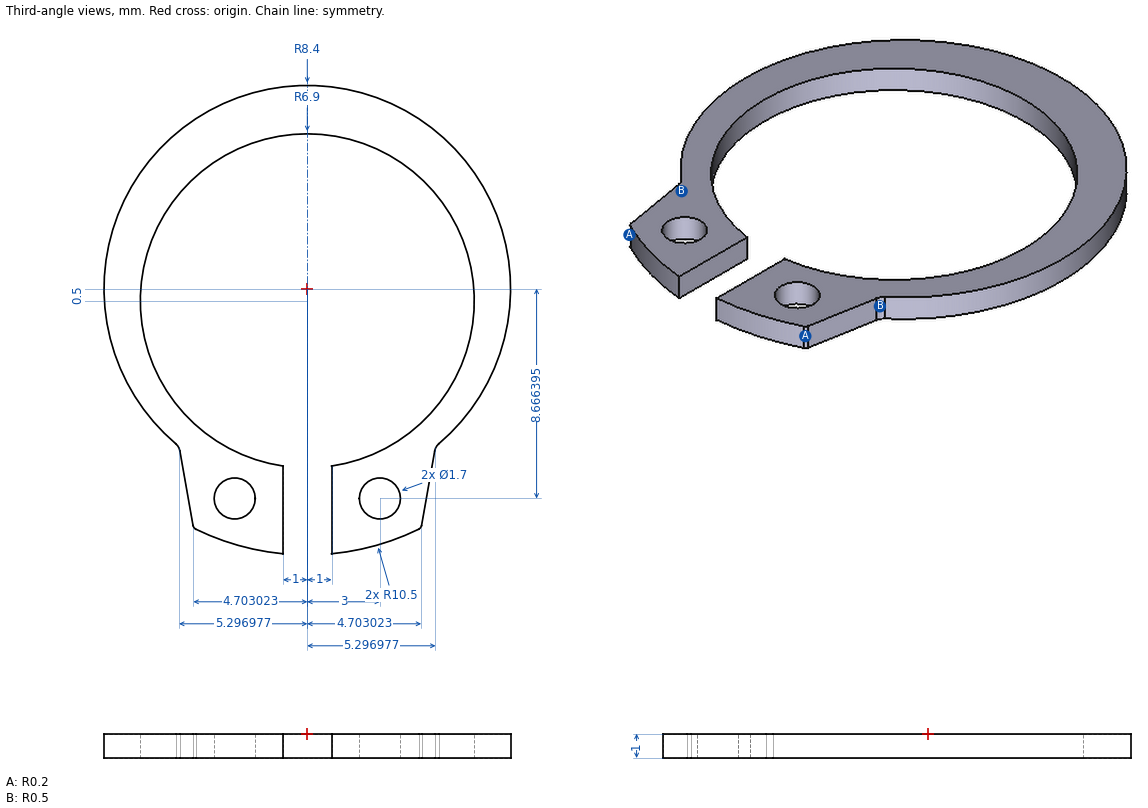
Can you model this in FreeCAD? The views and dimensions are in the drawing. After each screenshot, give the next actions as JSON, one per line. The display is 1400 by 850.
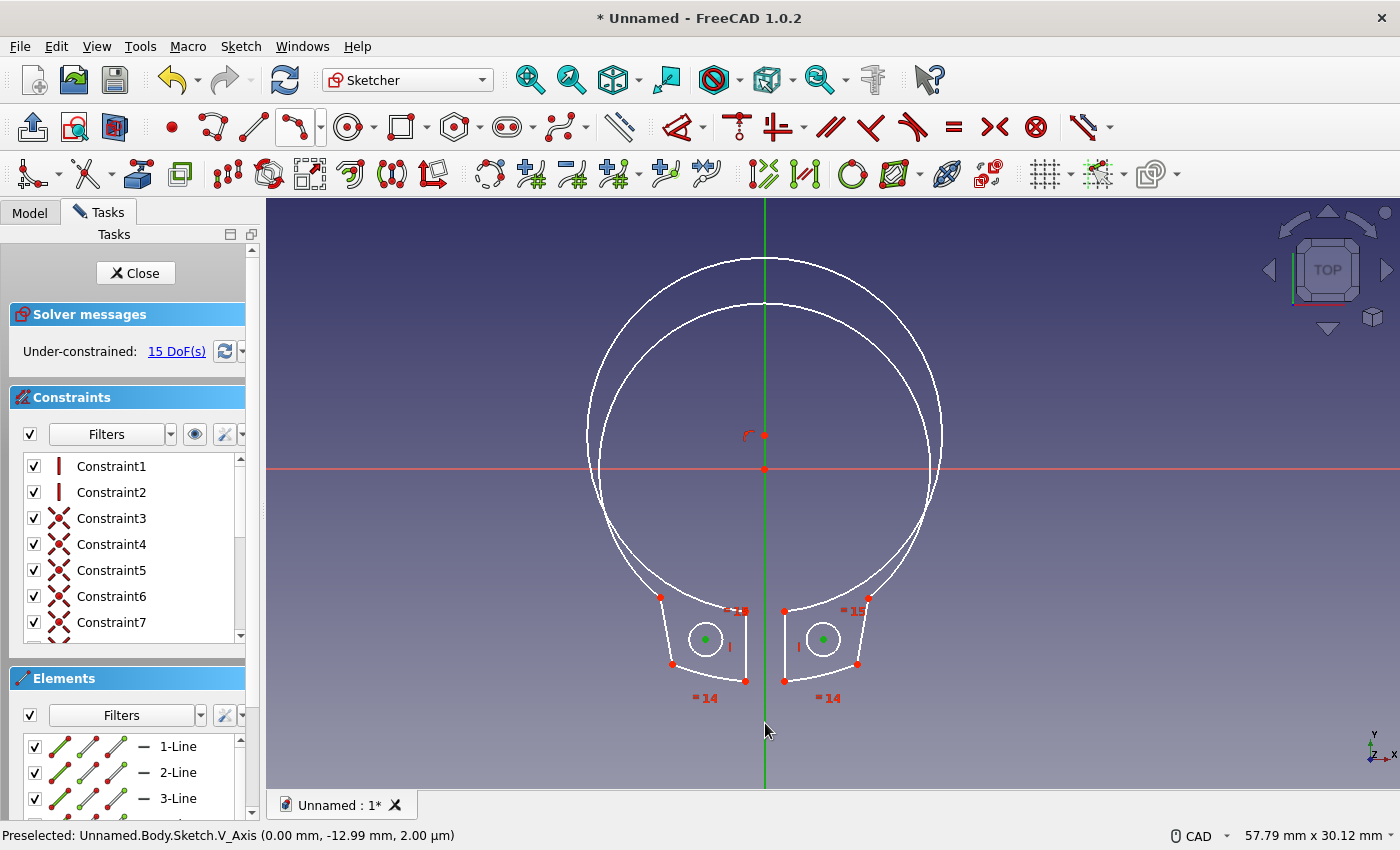
{"action": "left_click", "coordinate": [995, 128]}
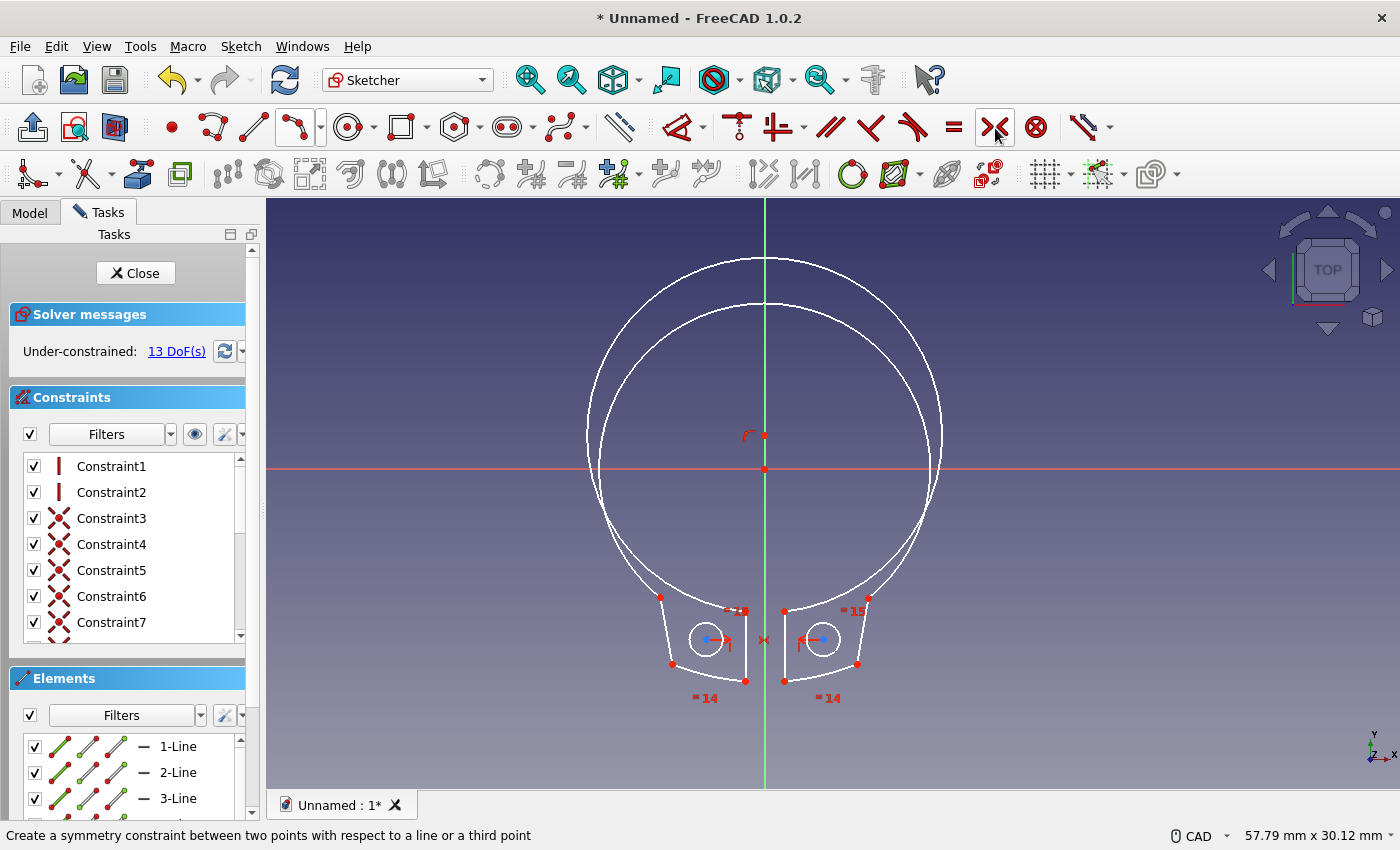
{"action": "left_click", "coordinate": [676, 128]}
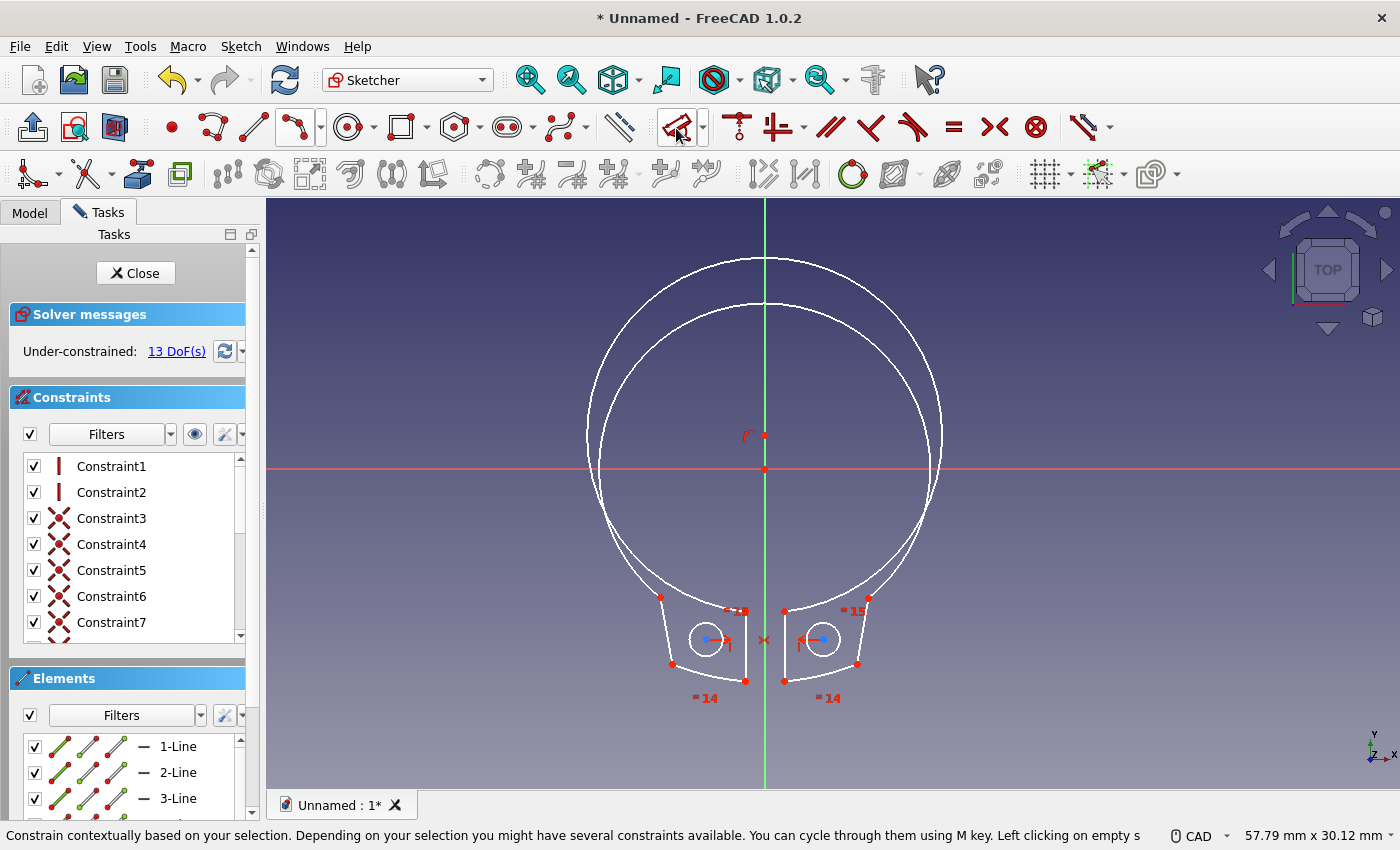
{"action": "left_click", "coordinate": [931, 372]}
{"action": "left_click", "coordinate": [961, 361]}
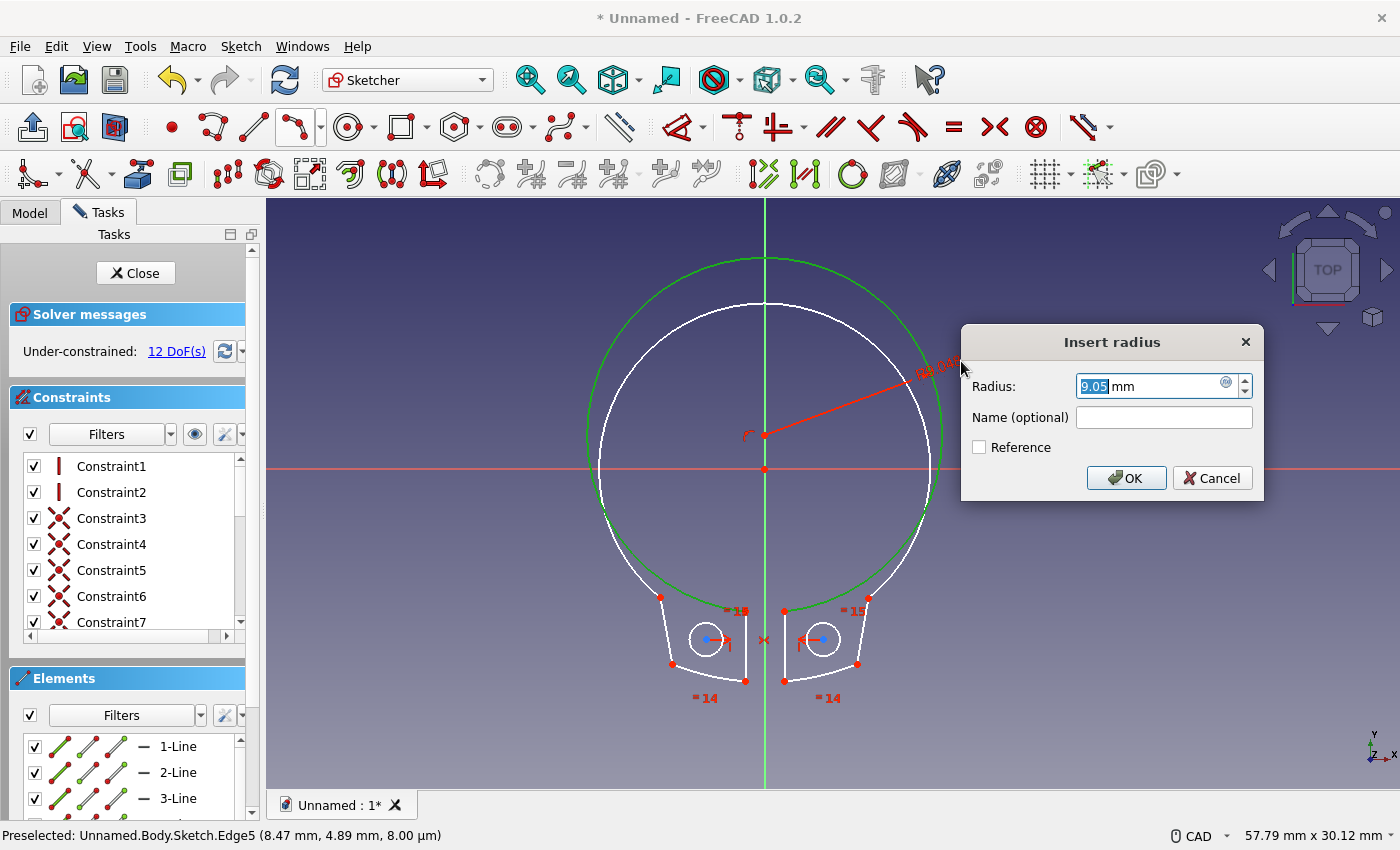
{"action": "type", "text": "6.9"}
{"action": "key", "text": "Return"}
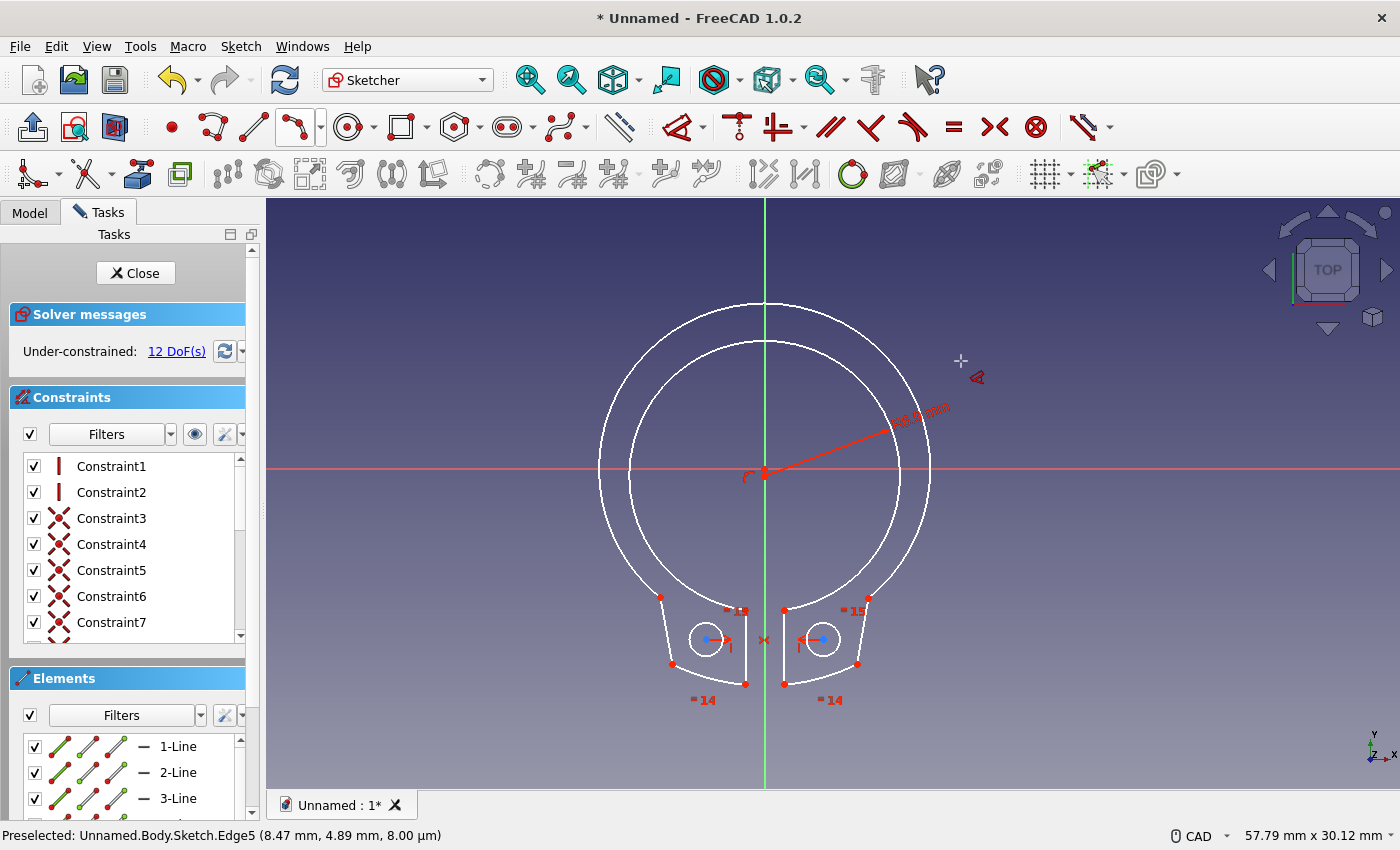
{"action": "left_click", "coordinate": [807, 681]}
{"action": "left_click", "coordinate": [813, 712]}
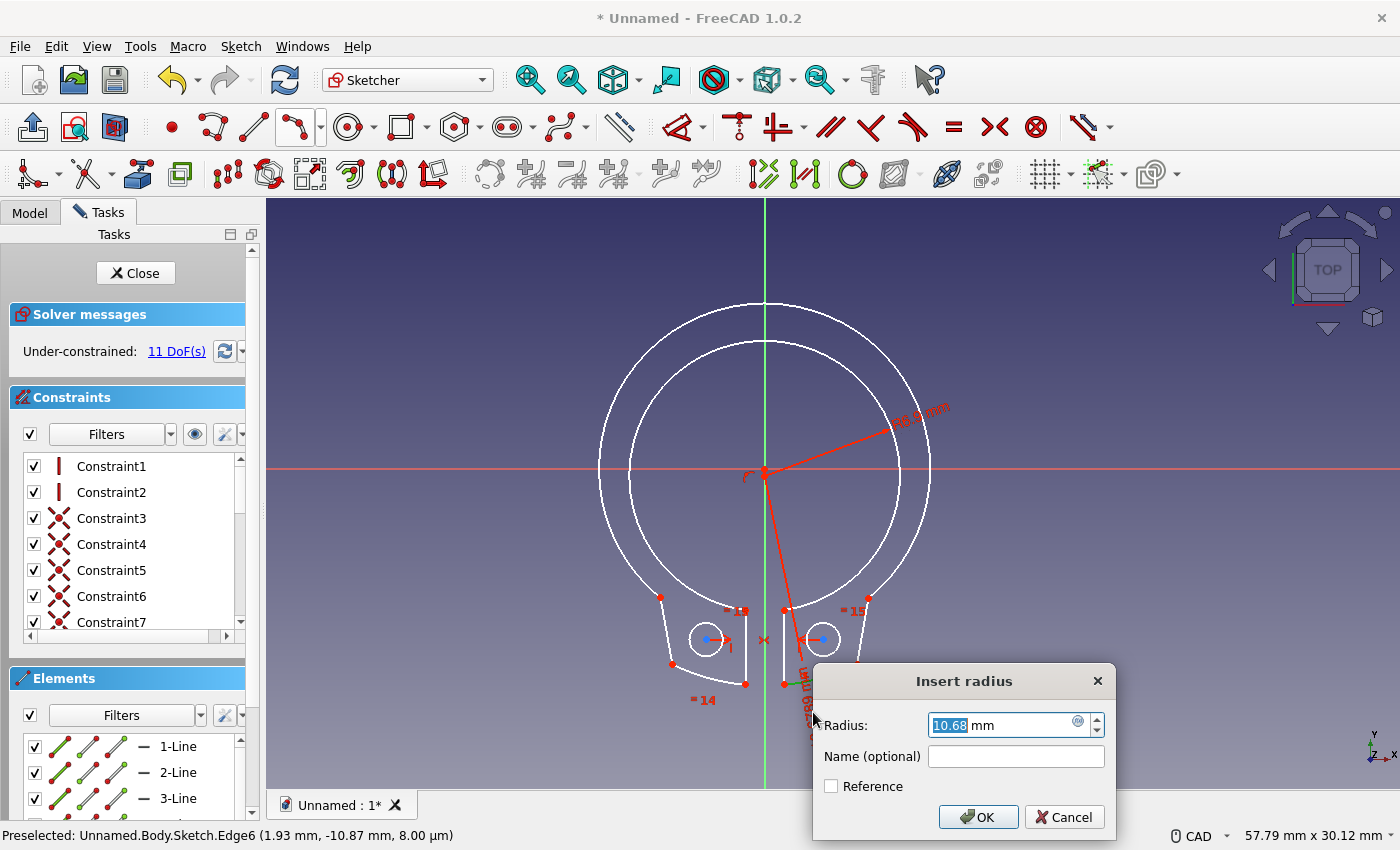
{"action": "type", "text": "10.5"}
{"action": "key", "text": "Return"}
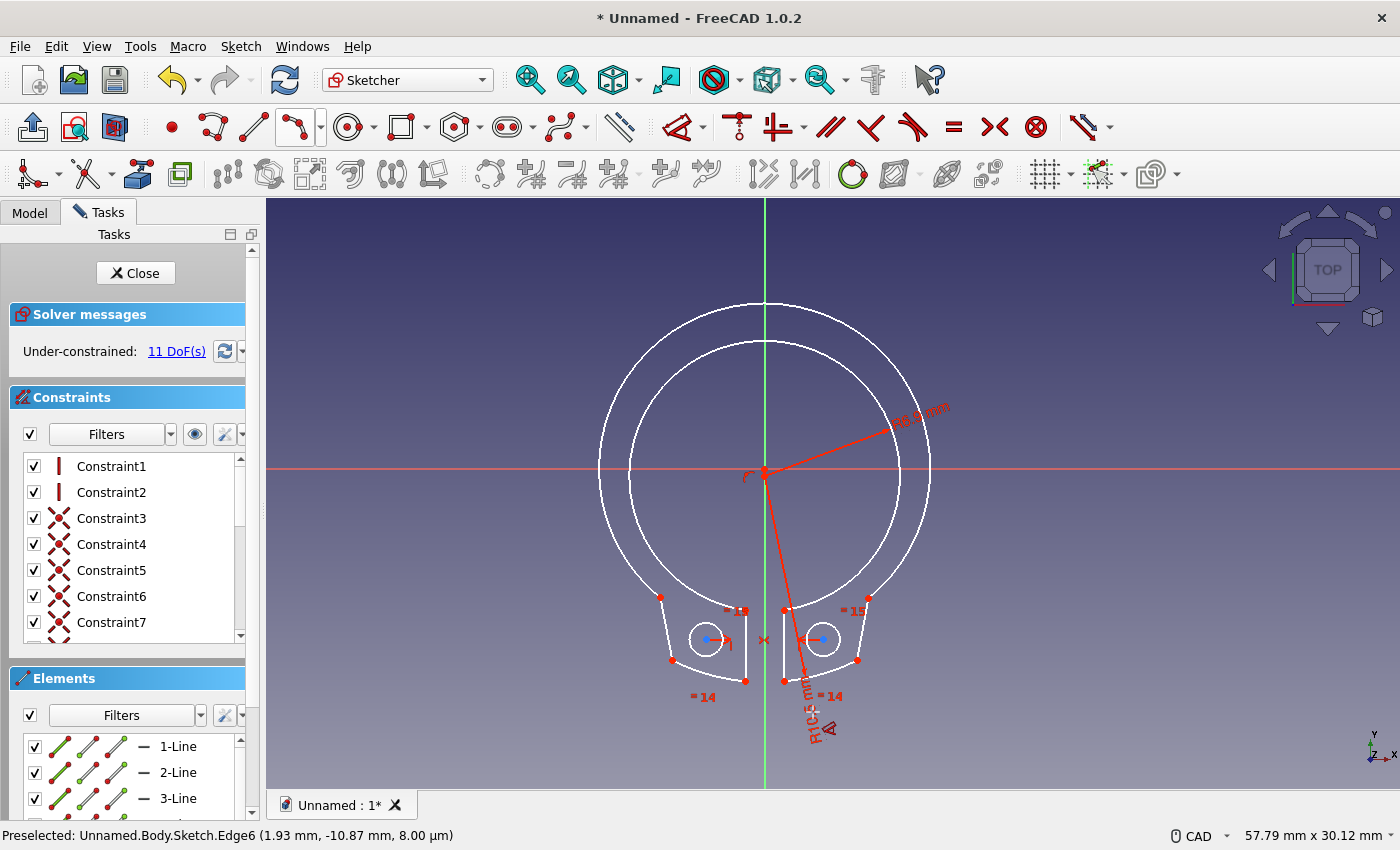
{"action": "left_click", "coordinate": [903, 378]}
{"action": "left_click", "coordinate": [962, 453]}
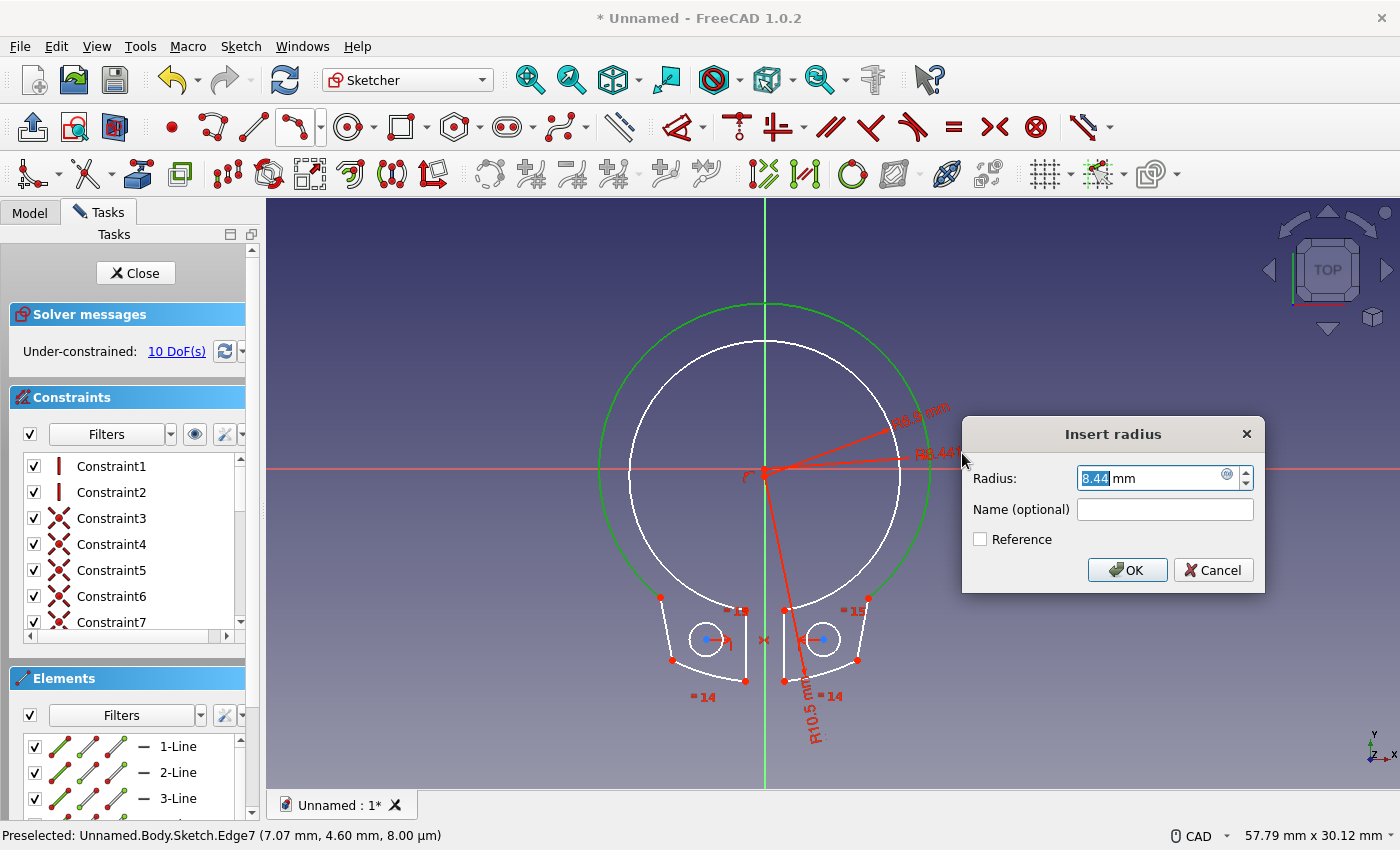
{"action": "type", "text": "8.4"}
{"action": "key", "text": "Return"}